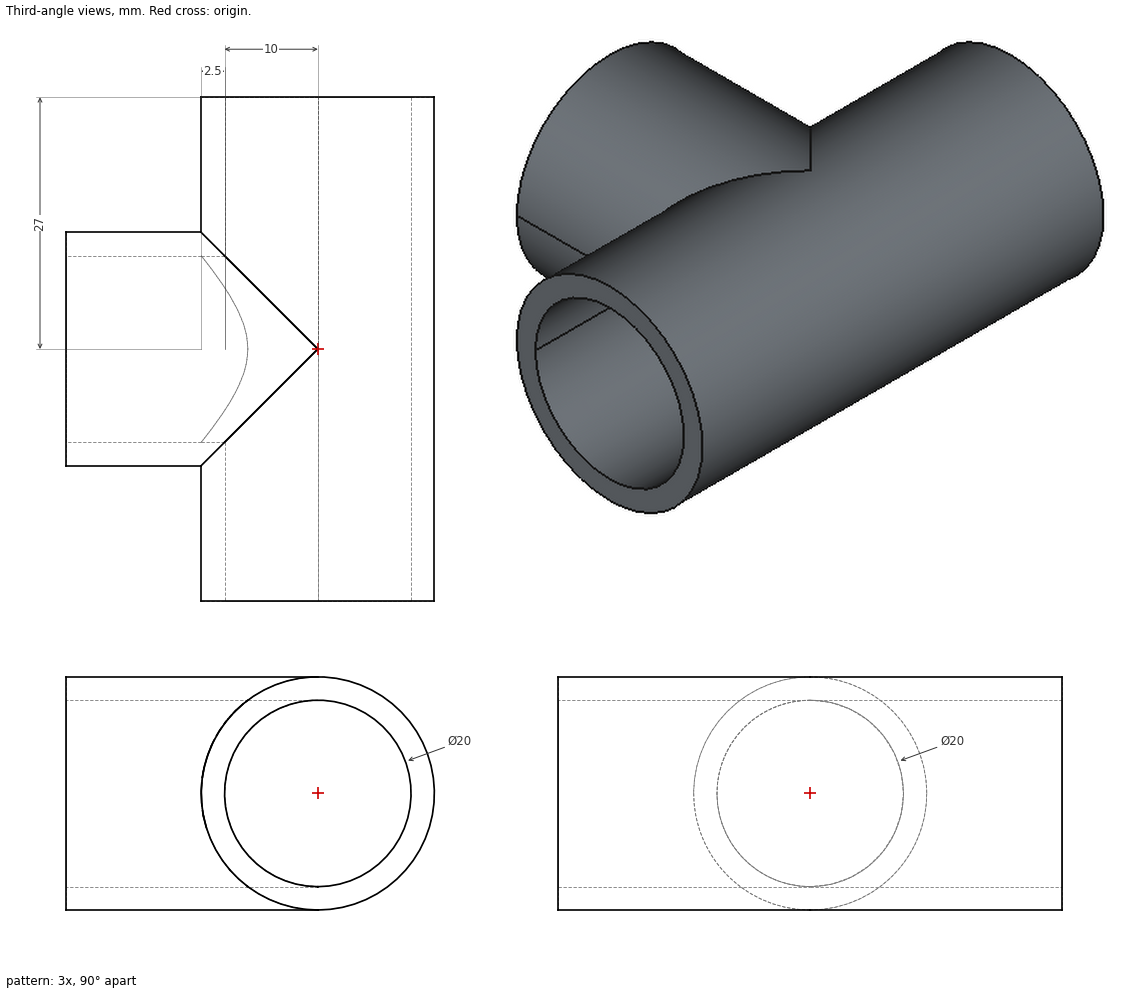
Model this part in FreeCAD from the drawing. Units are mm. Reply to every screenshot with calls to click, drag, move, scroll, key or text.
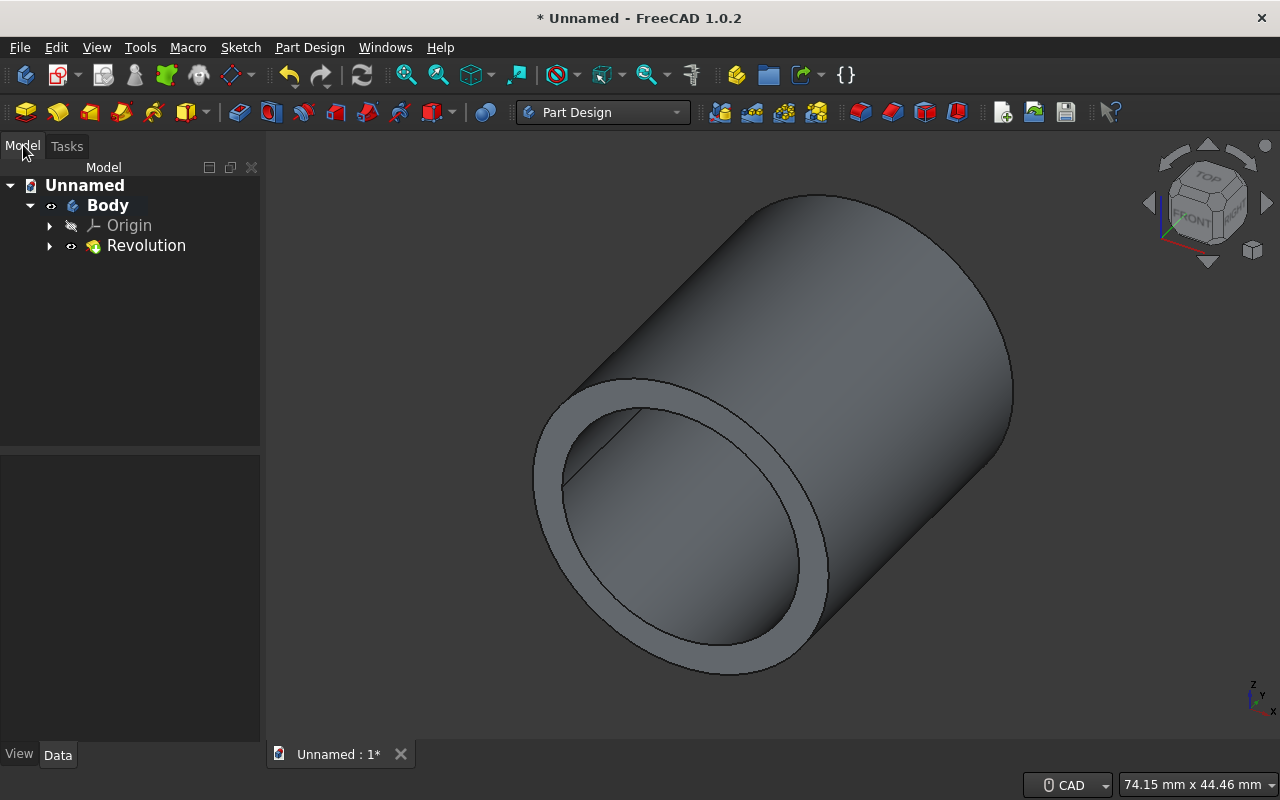
click(116, 246)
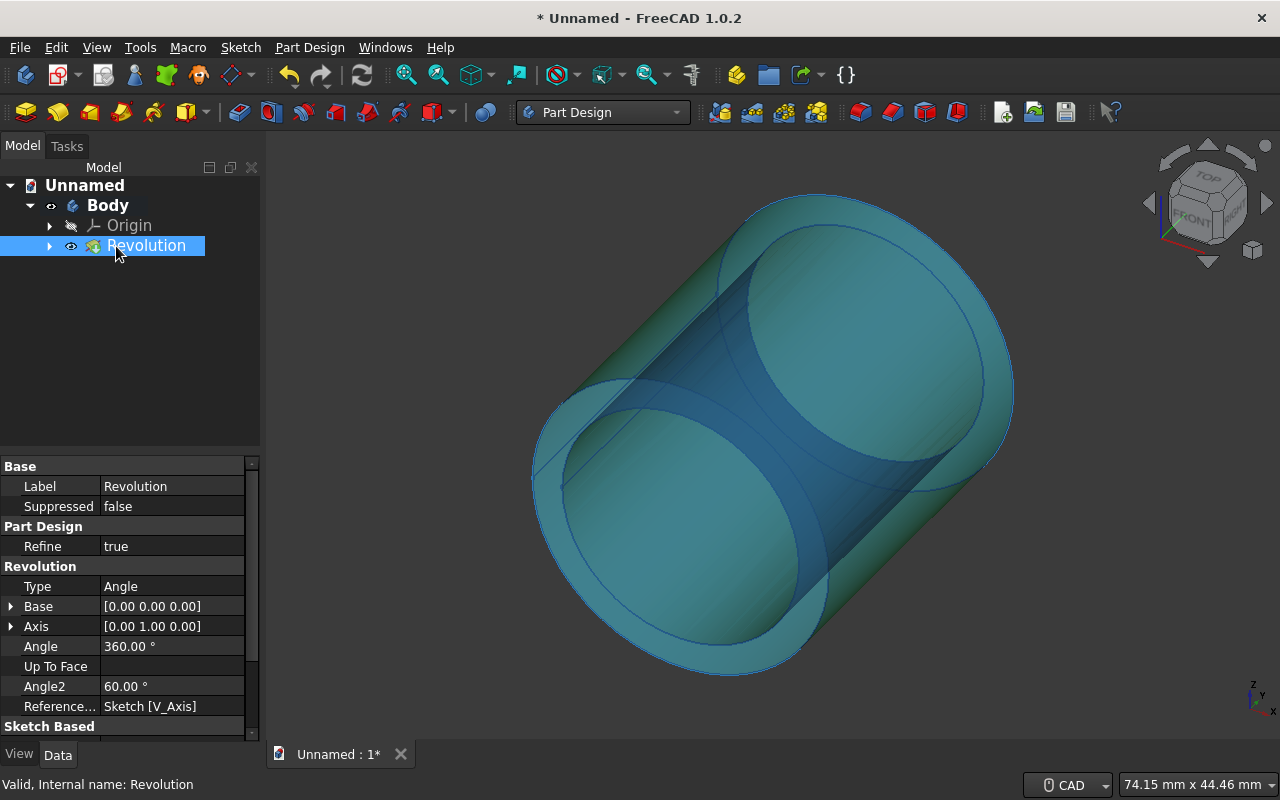
click(784, 112)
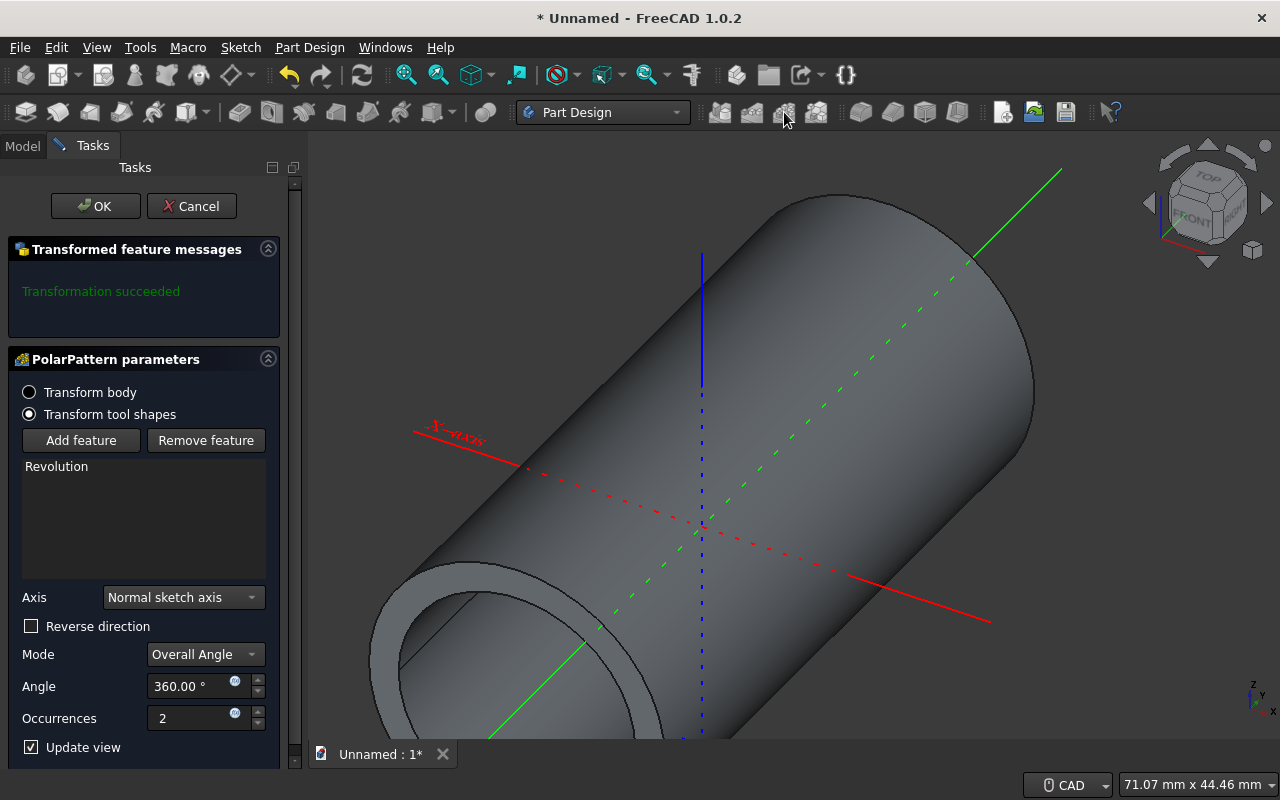
click(184, 598)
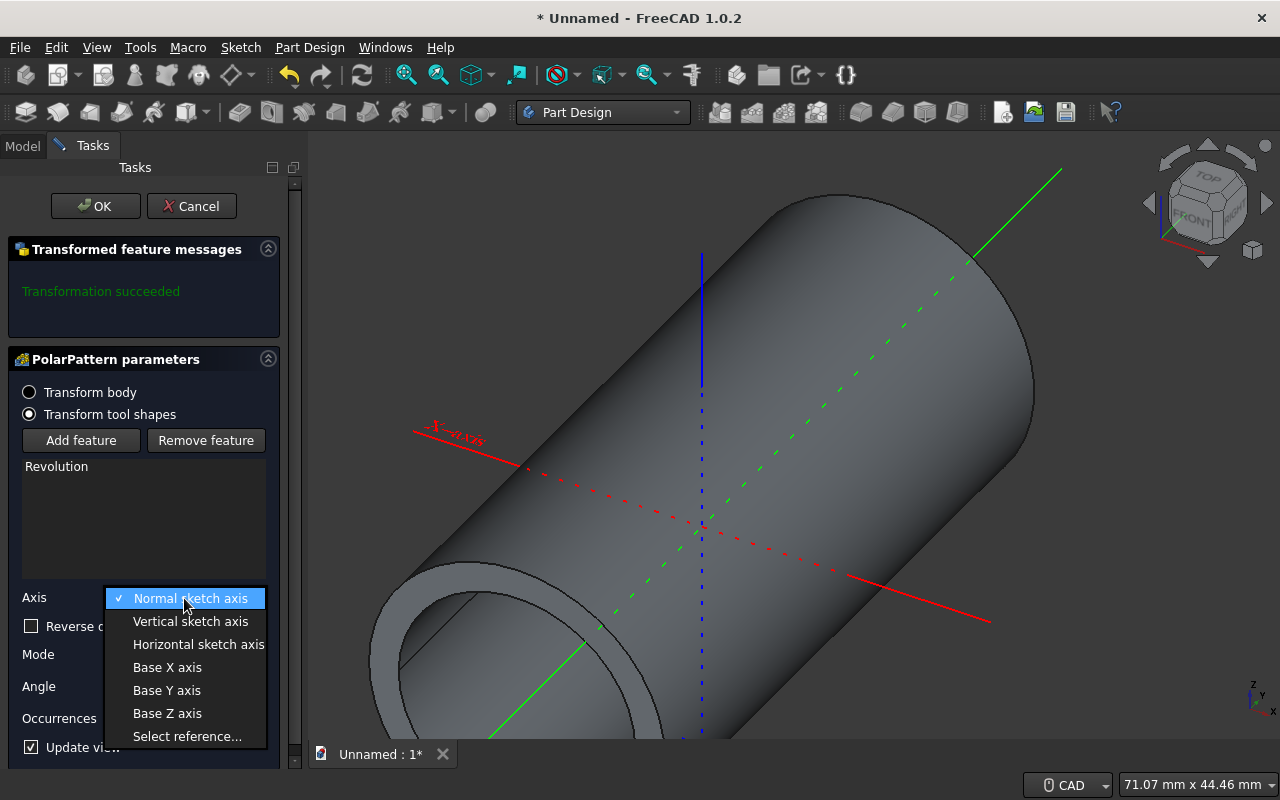
click(184, 714)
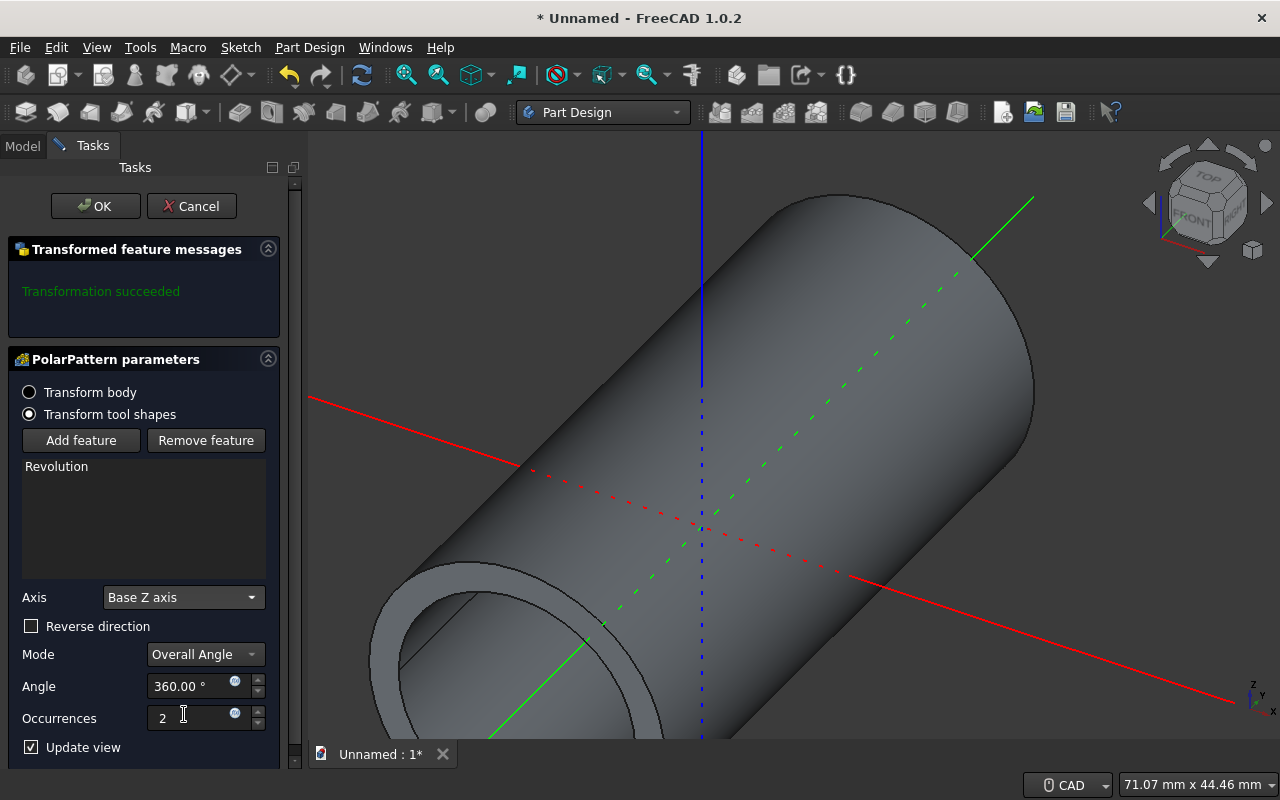
click(206, 654)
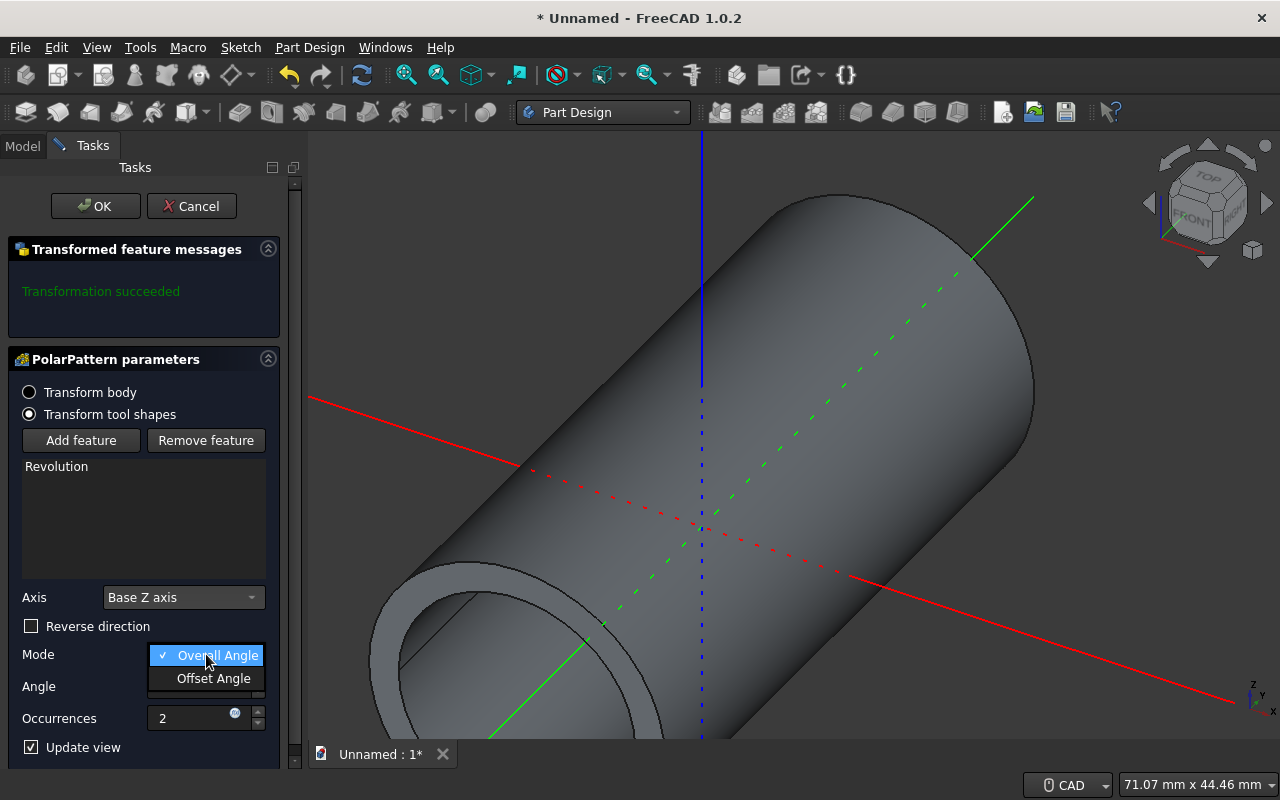
click(206, 678)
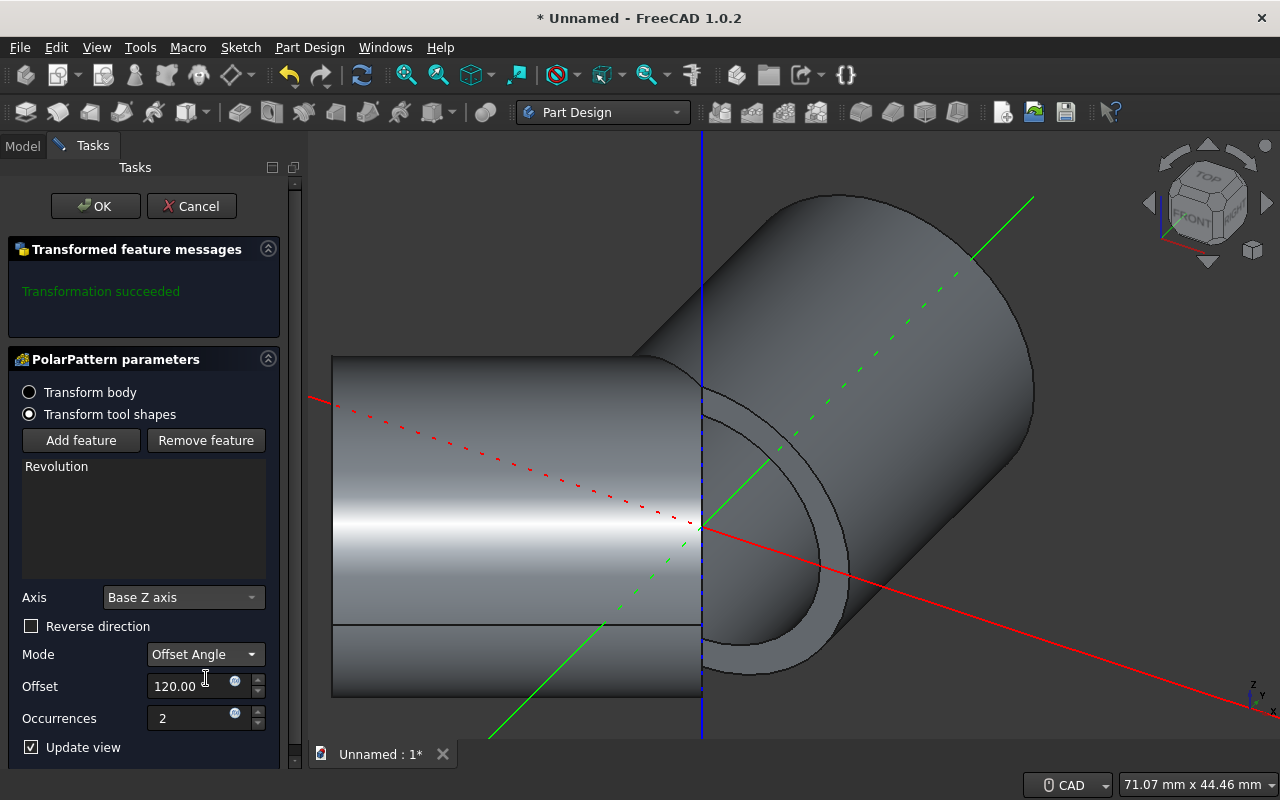
triple_click(198, 686)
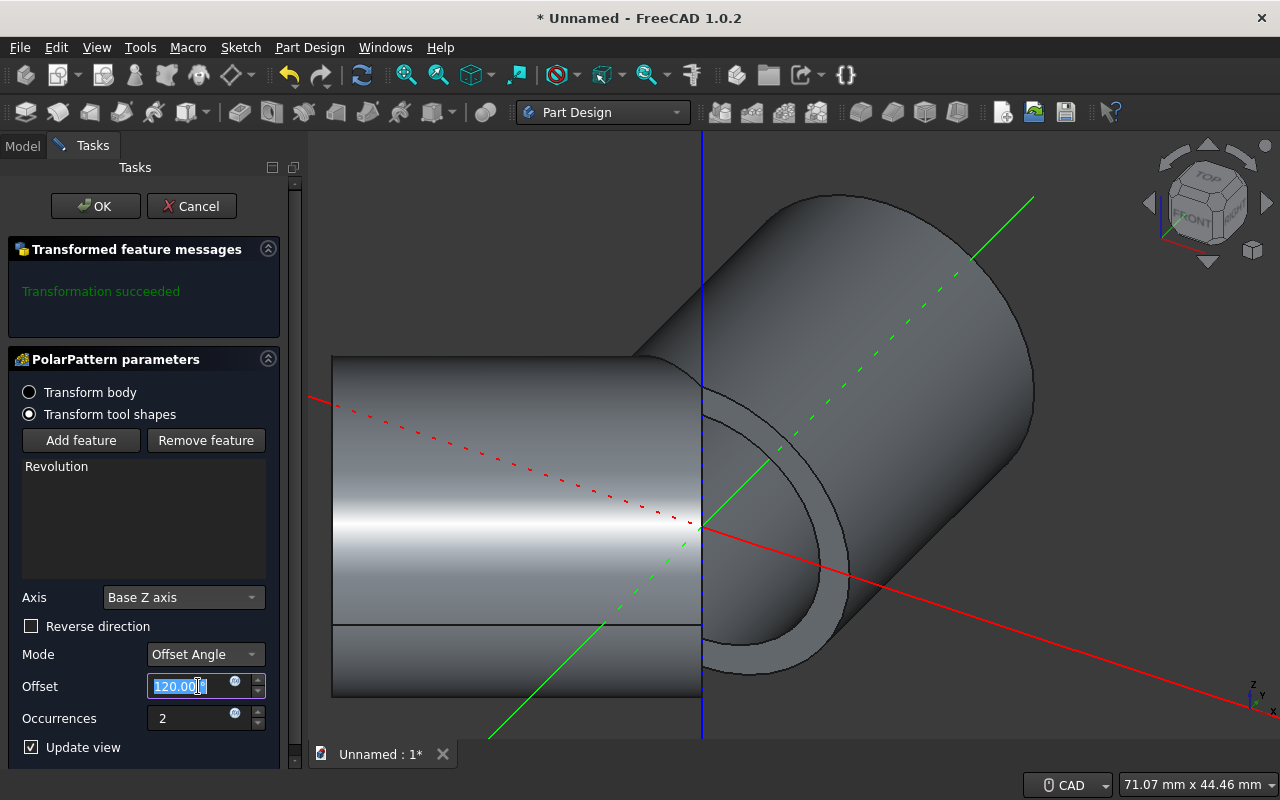
text(90)
key(Tab)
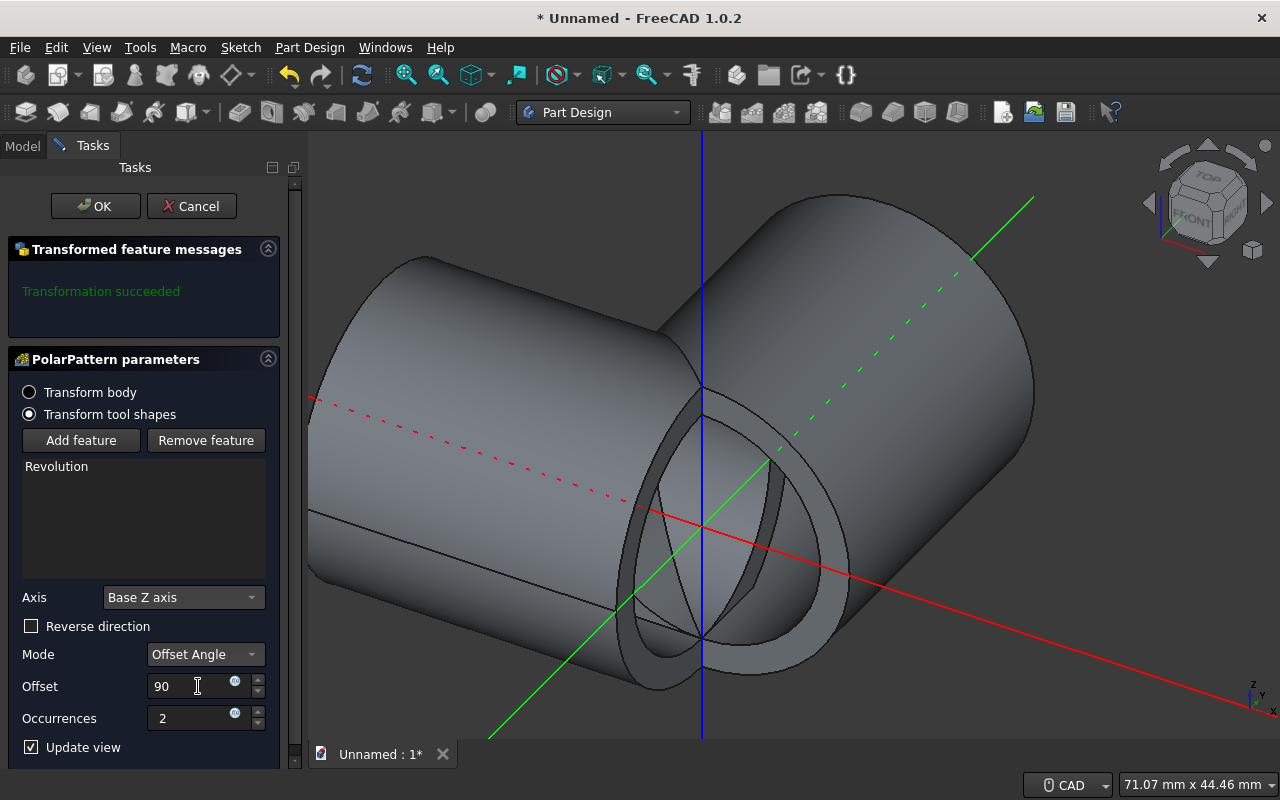
triple_click(198, 718)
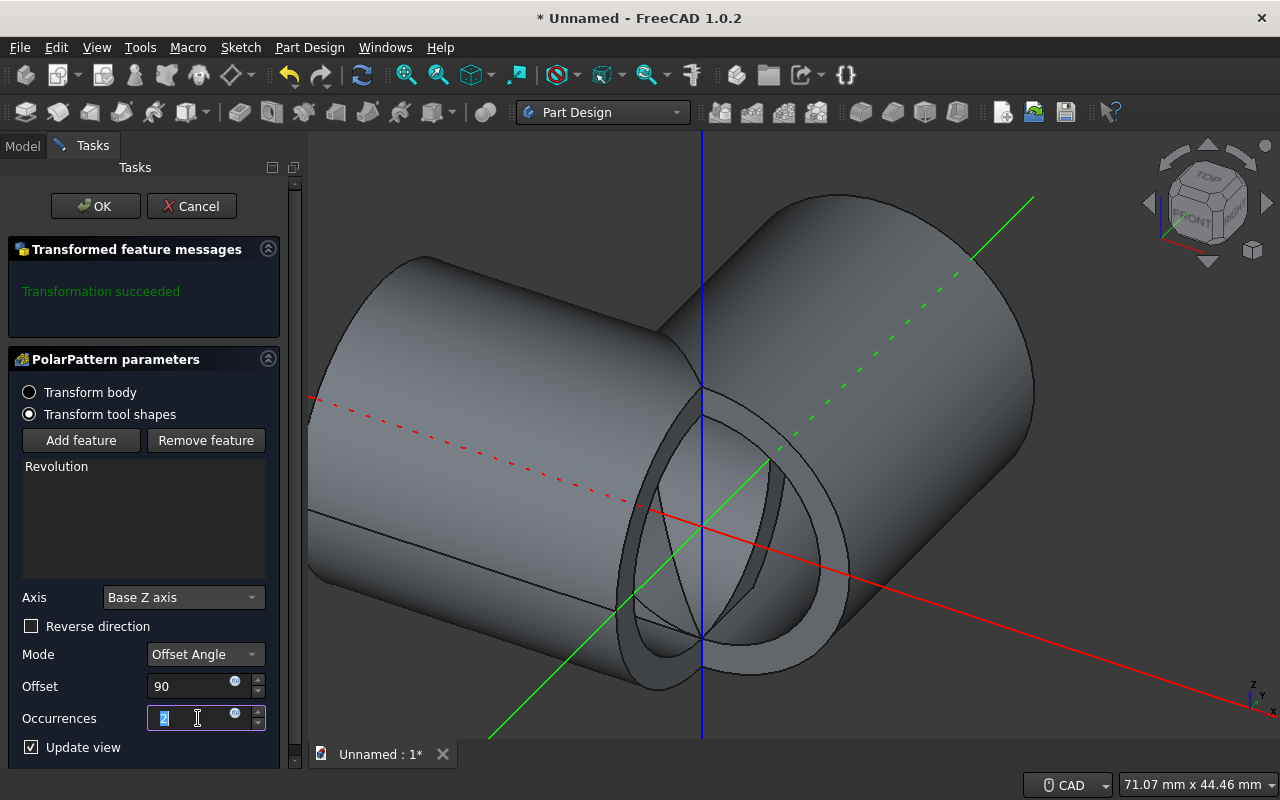
text(3)
key(Tab)